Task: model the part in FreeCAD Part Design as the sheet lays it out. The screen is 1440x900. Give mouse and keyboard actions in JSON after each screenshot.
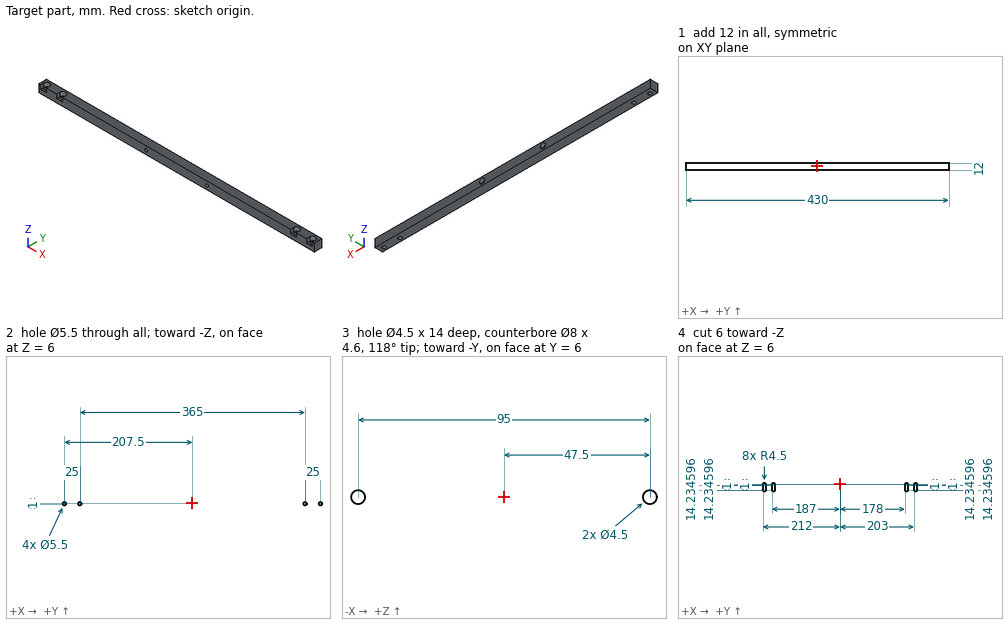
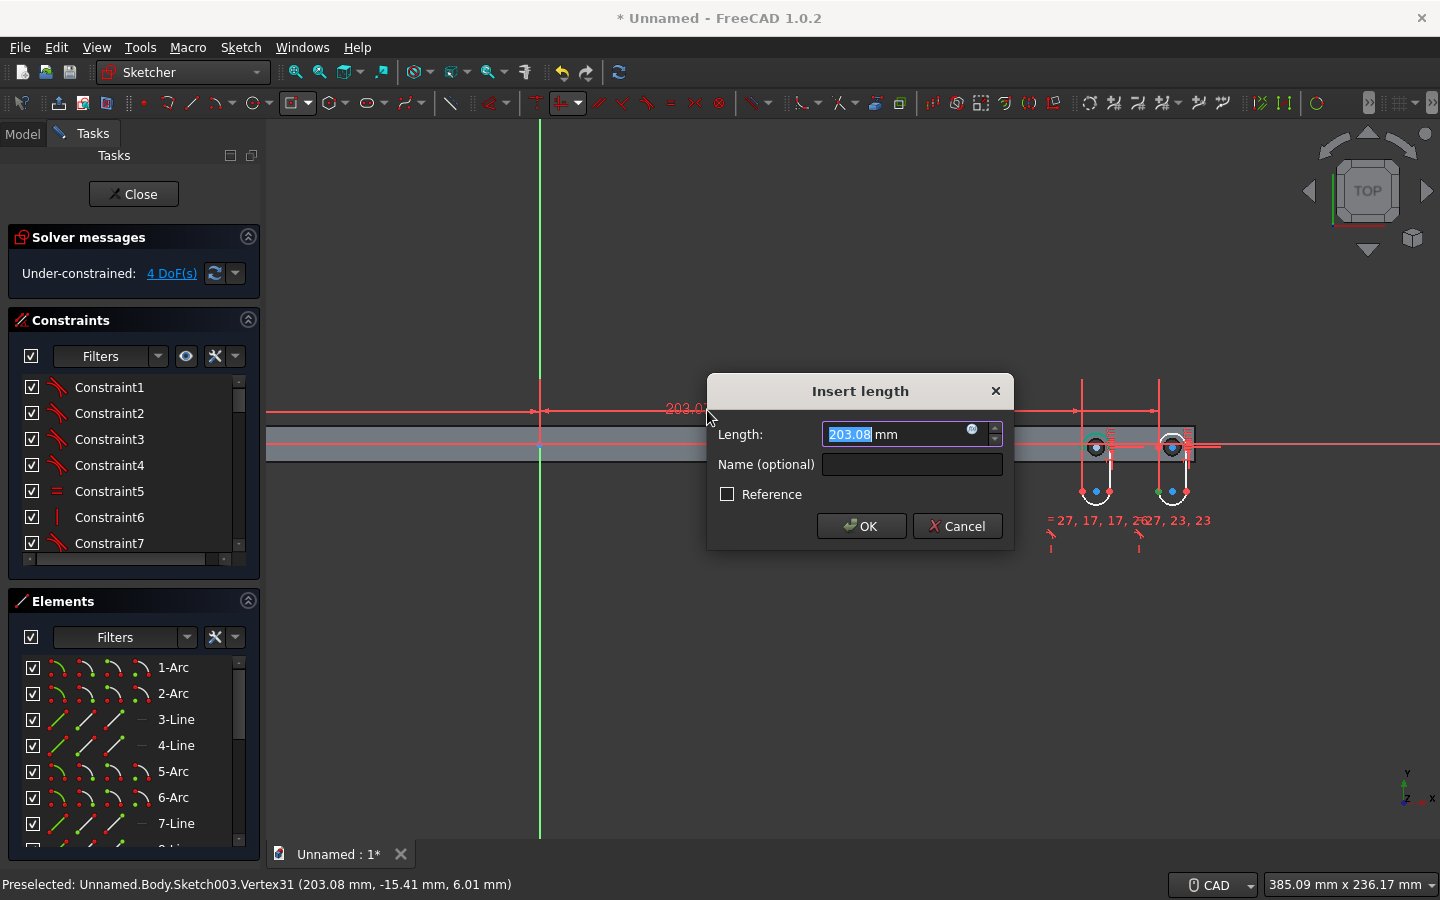
{"action": "type", "text": "203"}
{"action": "key", "text": "Return"}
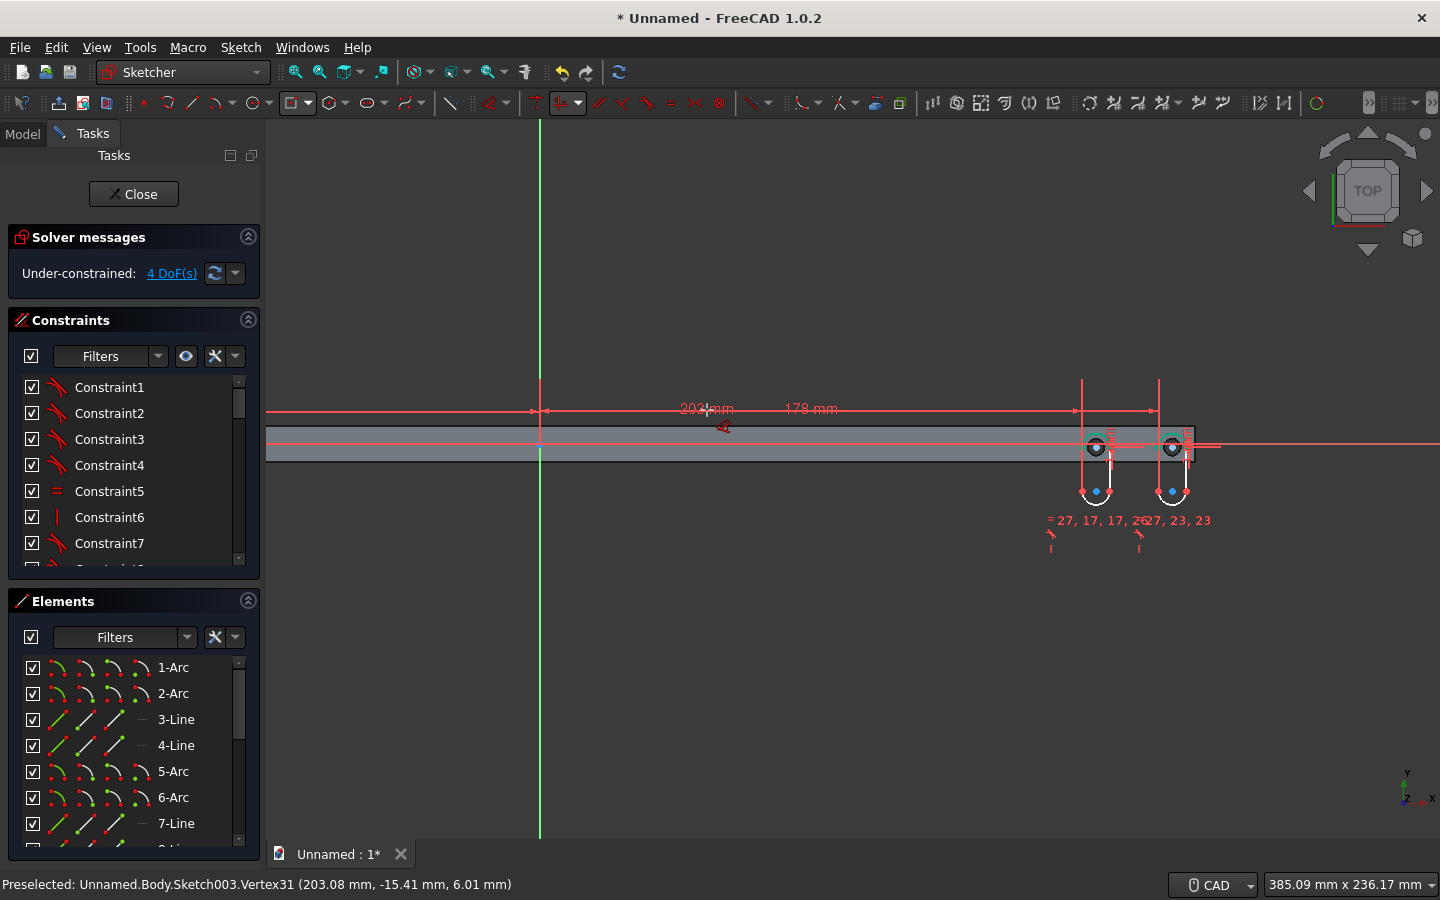
{"action": "scroll", "coordinate": [1082, 491], "scroll_direction": "down", "scroll_amount": 3}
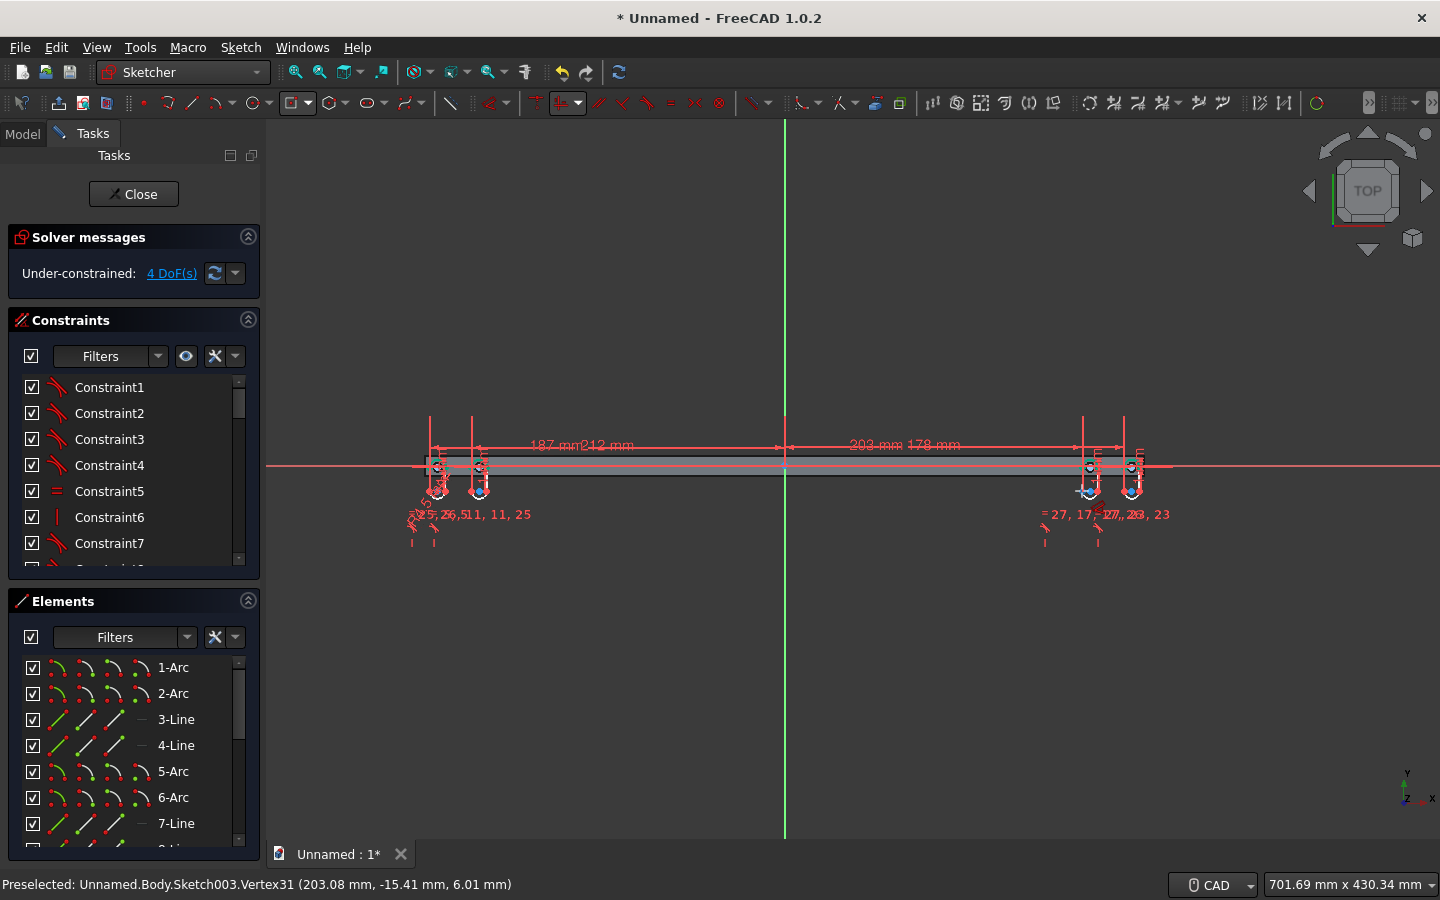
{"action": "scroll", "coordinate": [430, 484], "scroll_direction": "up", "scroll_amount": 4}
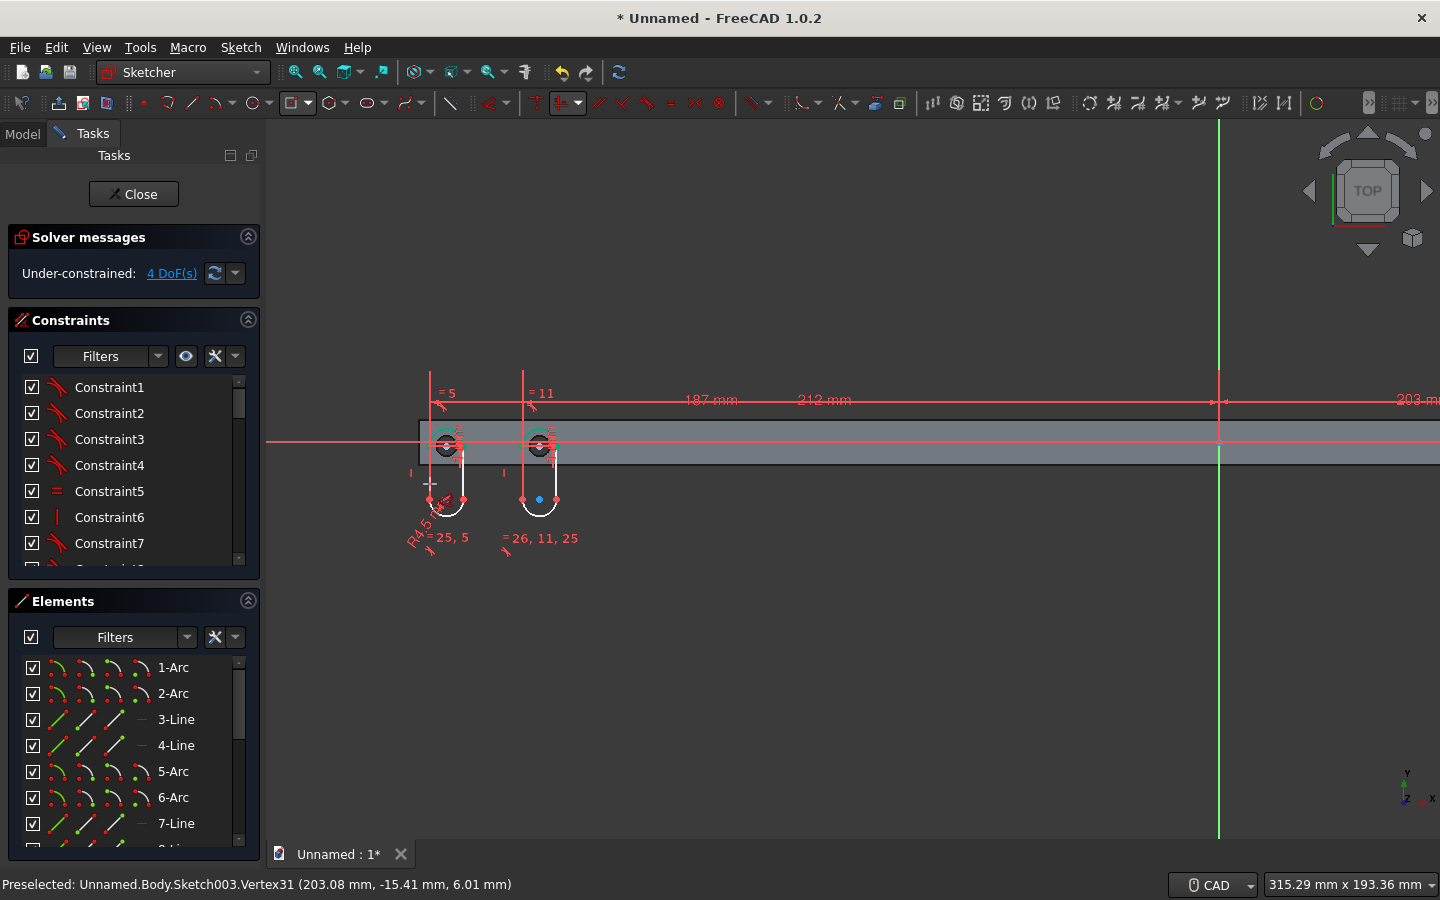
{"action": "left_click", "coordinate": [430, 483]}
{"action": "left_click", "coordinate": [396, 473]}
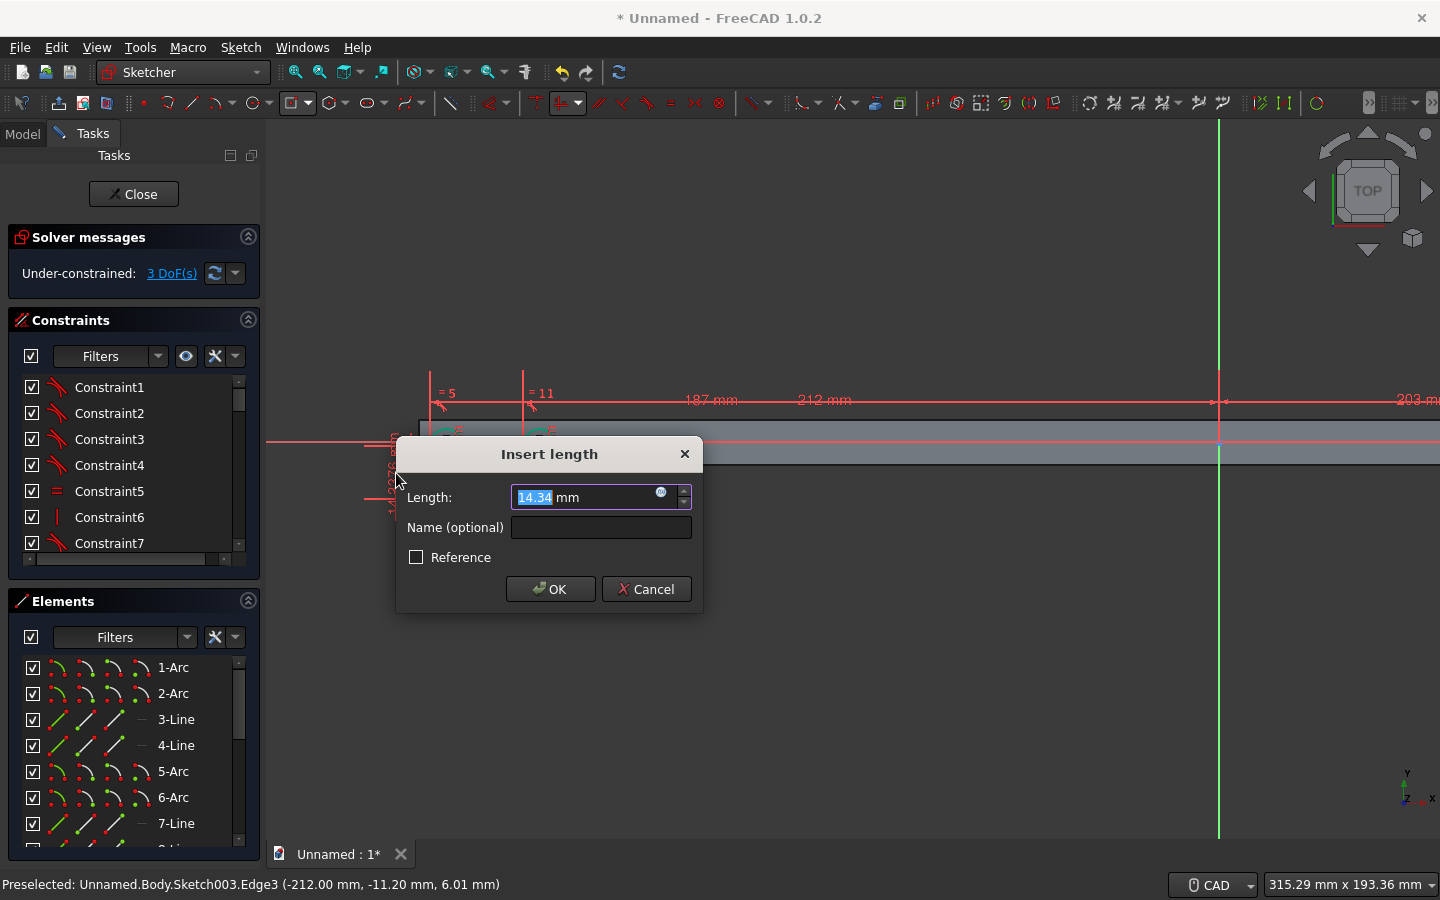
{"action": "type", "text": "14.234596"}
{"action": "key", "text": "Return"}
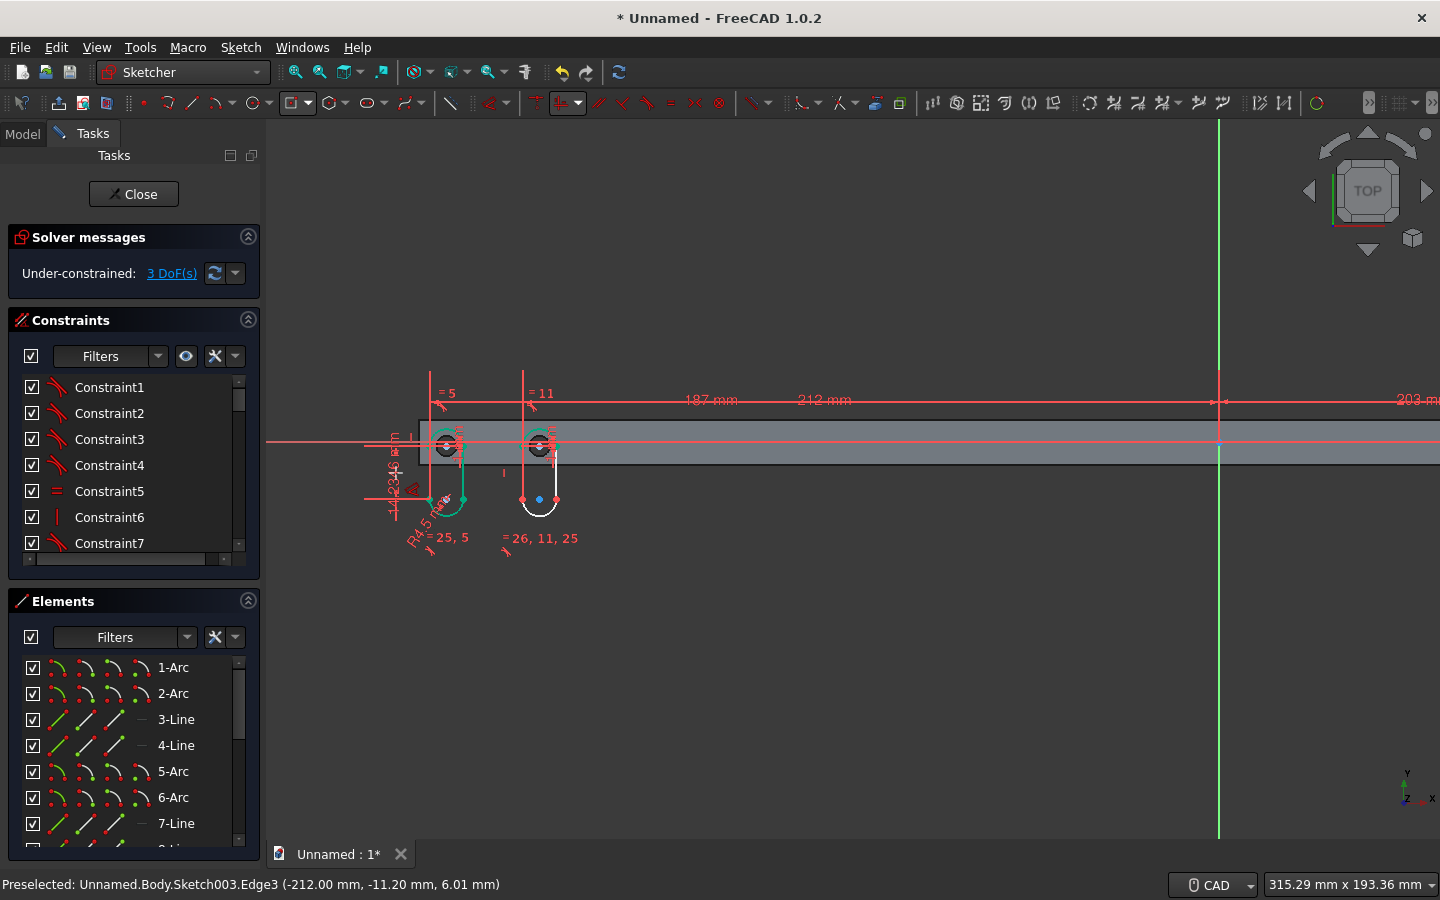
{"action": "left_click", "coordinate": [523, 484]}
{"action": "left_click", "coordinate": [489, 473]}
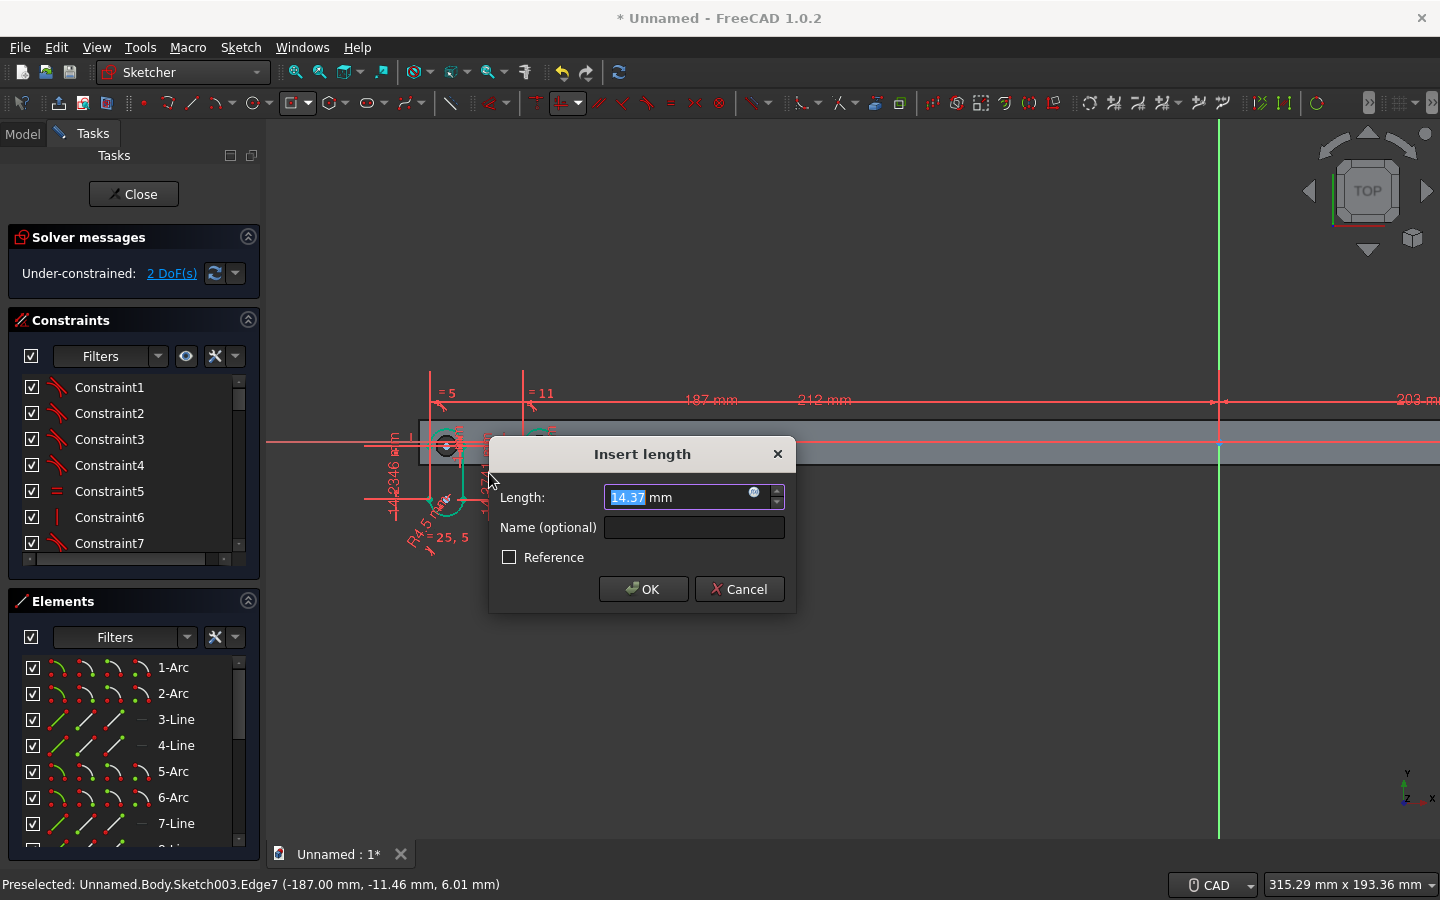
{"action": "type", "text": "14.234596"}
{"action": "key", "text": "Return"}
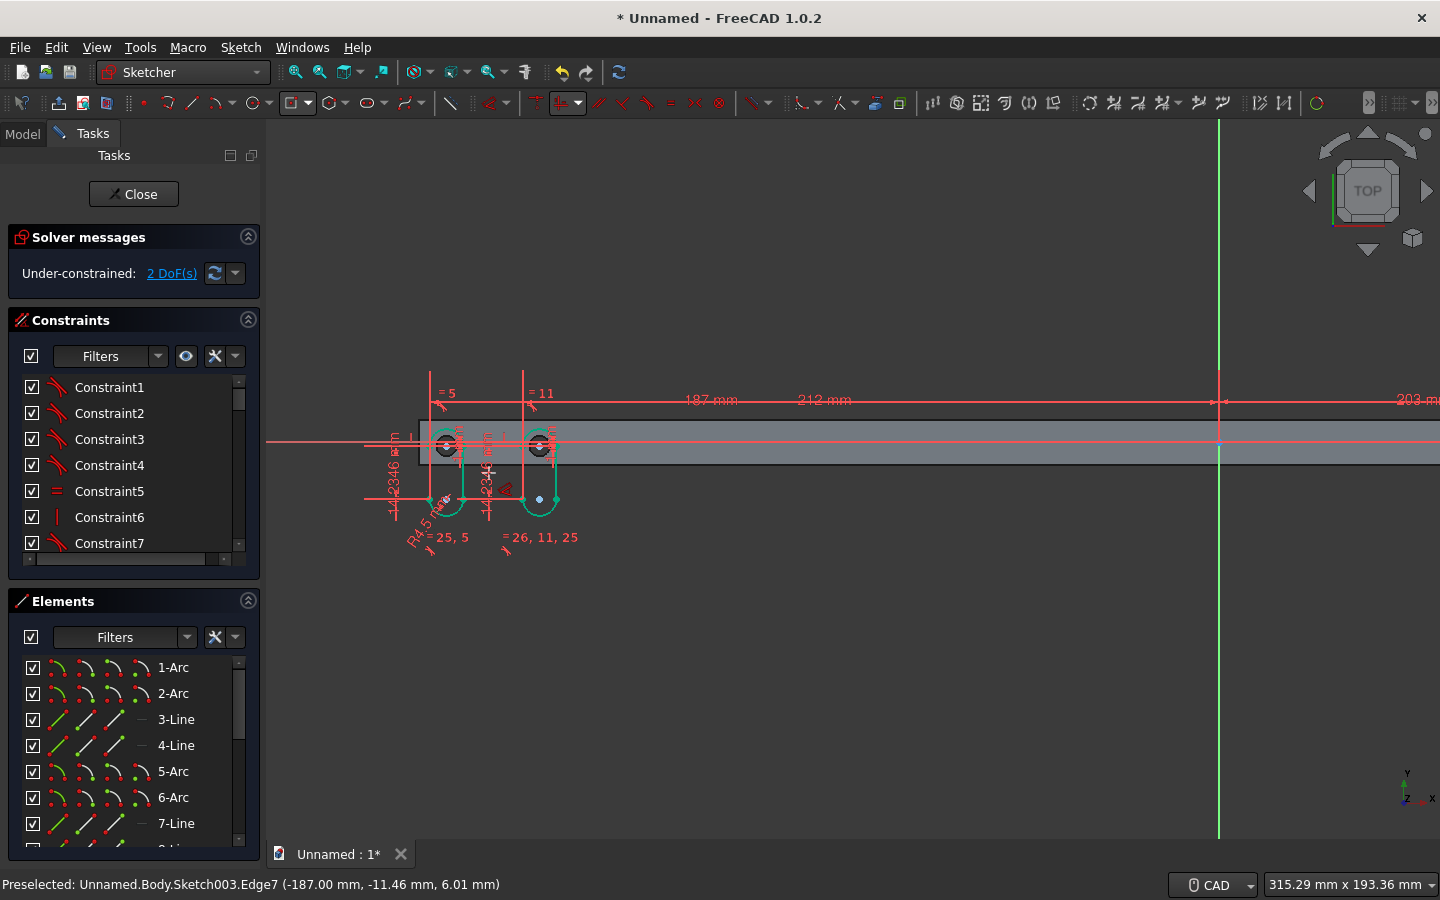
{"action": "scroll", "coordinate": [430, 484], "scroll_direction": "down", "scroll_amount": 4}